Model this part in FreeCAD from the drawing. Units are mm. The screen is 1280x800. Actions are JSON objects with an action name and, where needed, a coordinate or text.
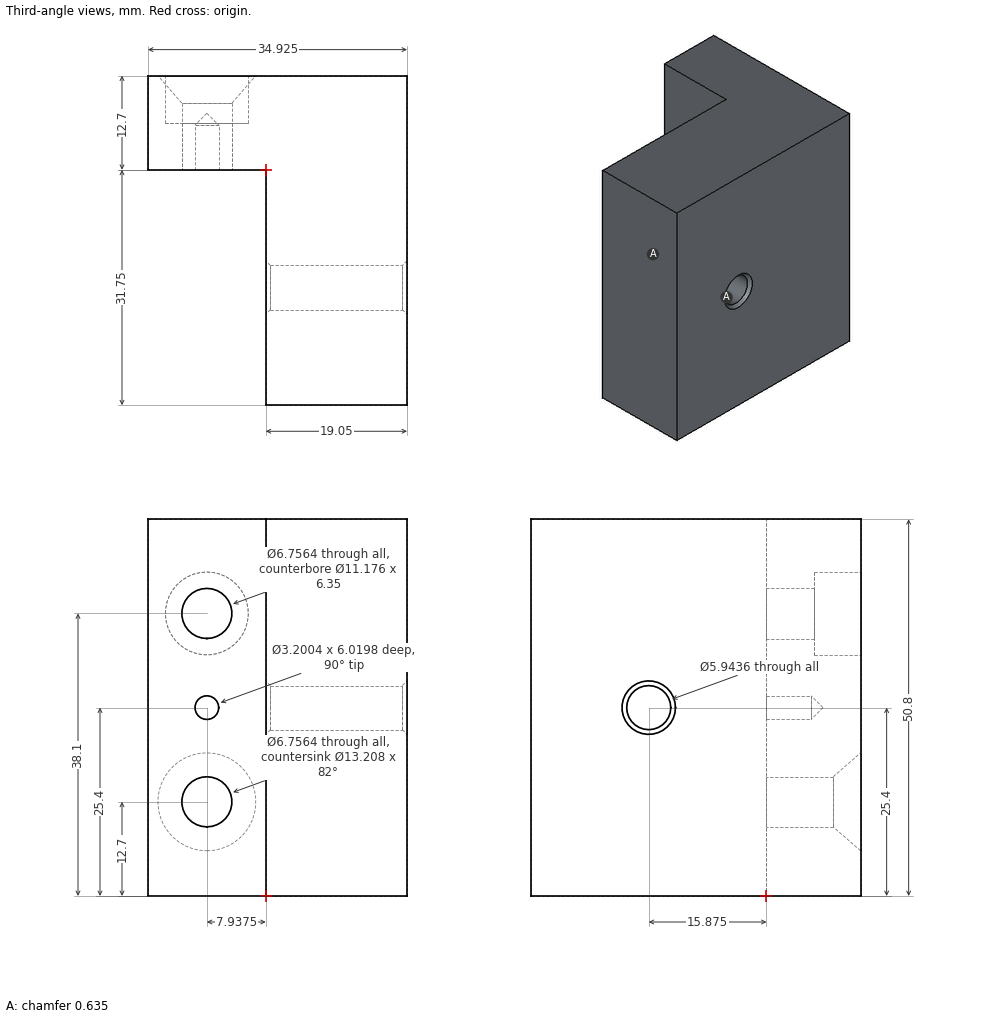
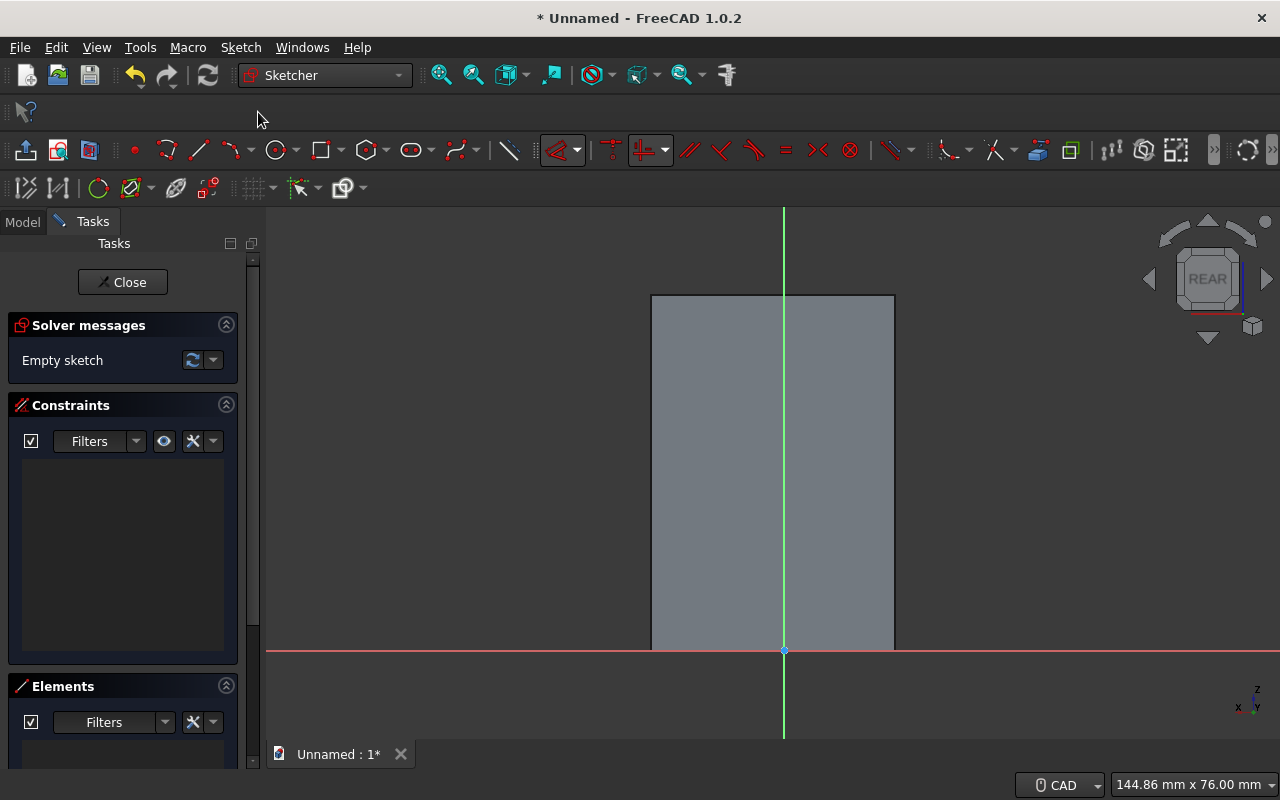
{"action": "scroll", "coordinate": [893, 665], "scroll_direction": "up", "scroll_amount": 5}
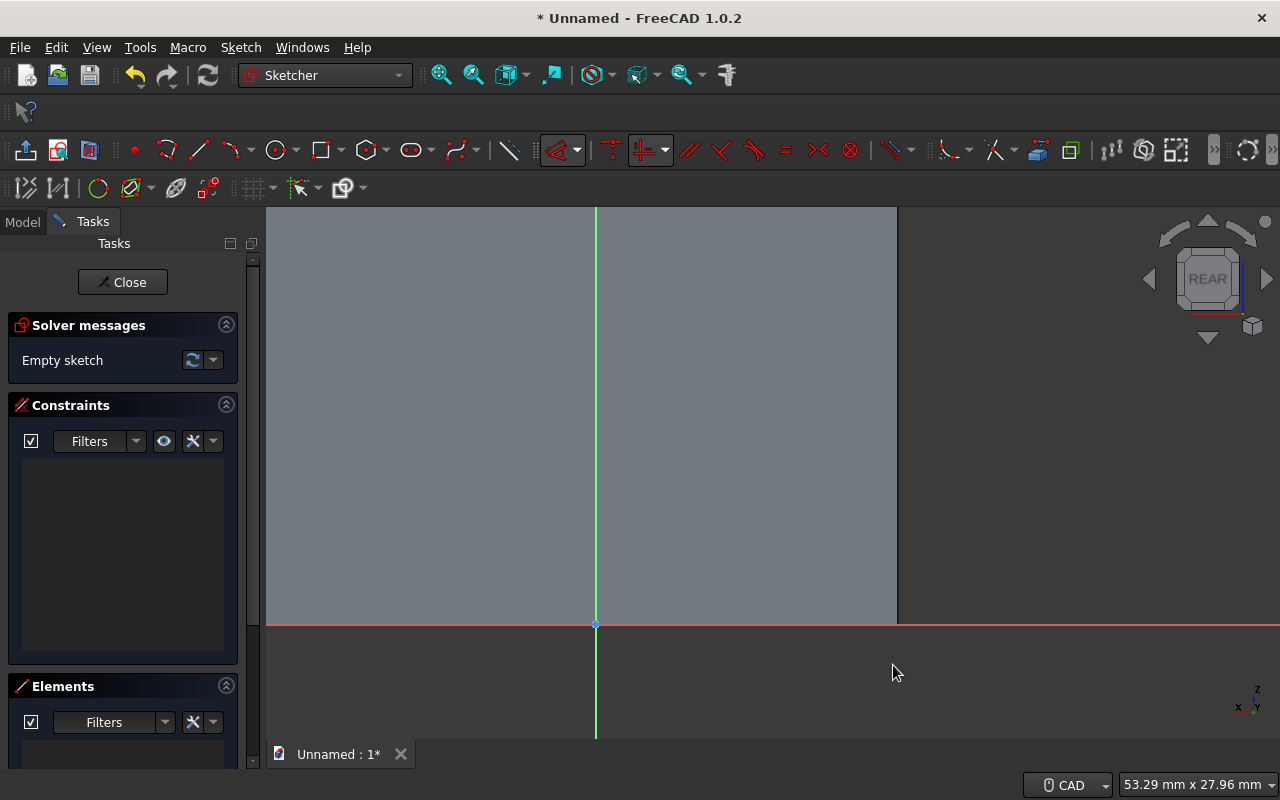
{"action": "left_click", "coordinate": [276, 150]}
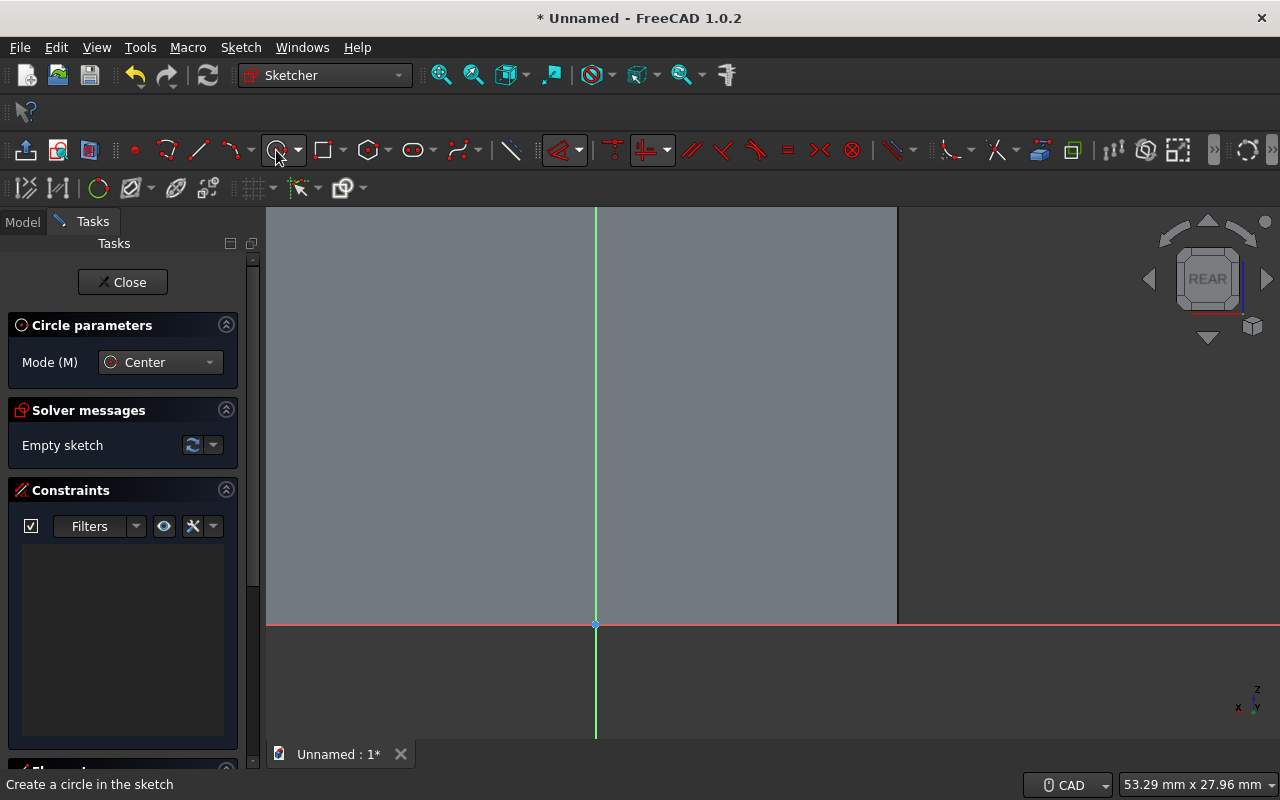
{"action": "left_click", "coordinate": [747, 383]}
{"action": "mouse_move", "coordinate": [792, 338]}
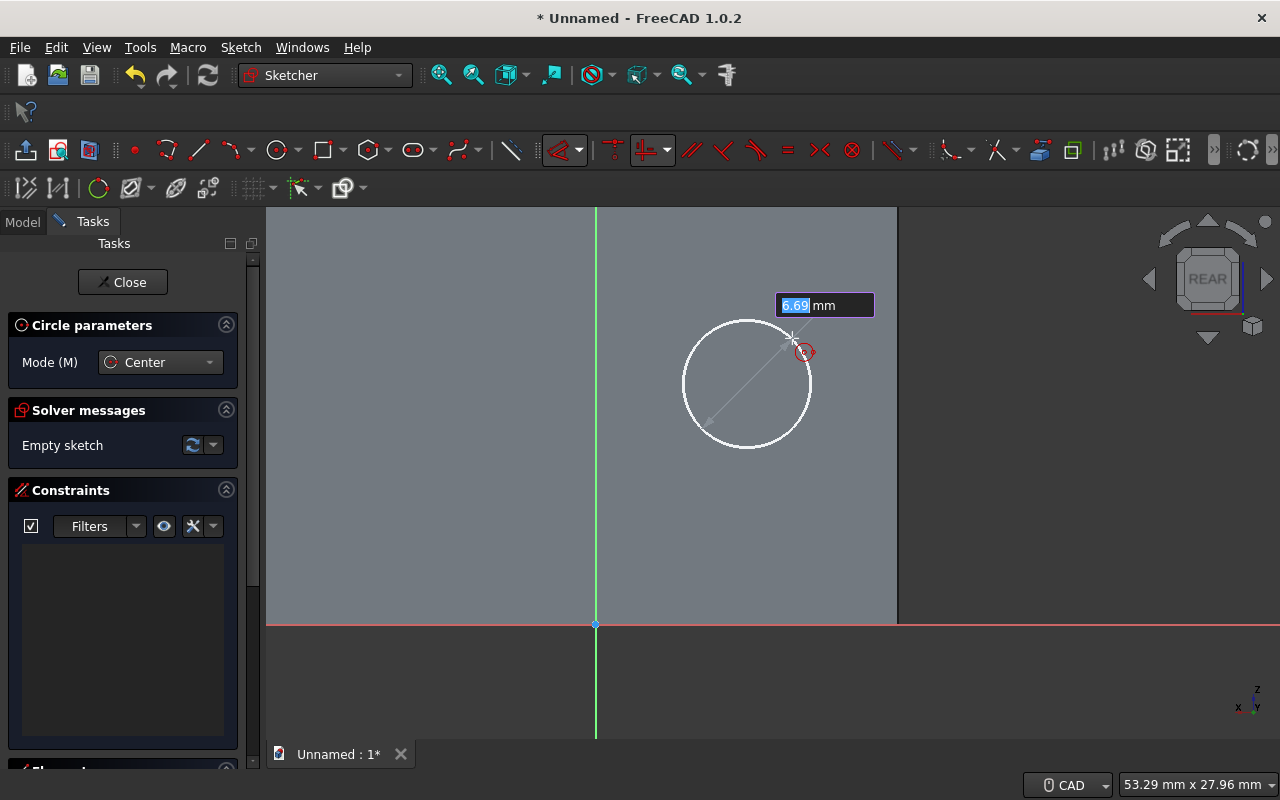
{"action": "type", "text": "6.7564"}
{"action": "key", "text": "Return"}
{"action": "key", "text": "Escape"}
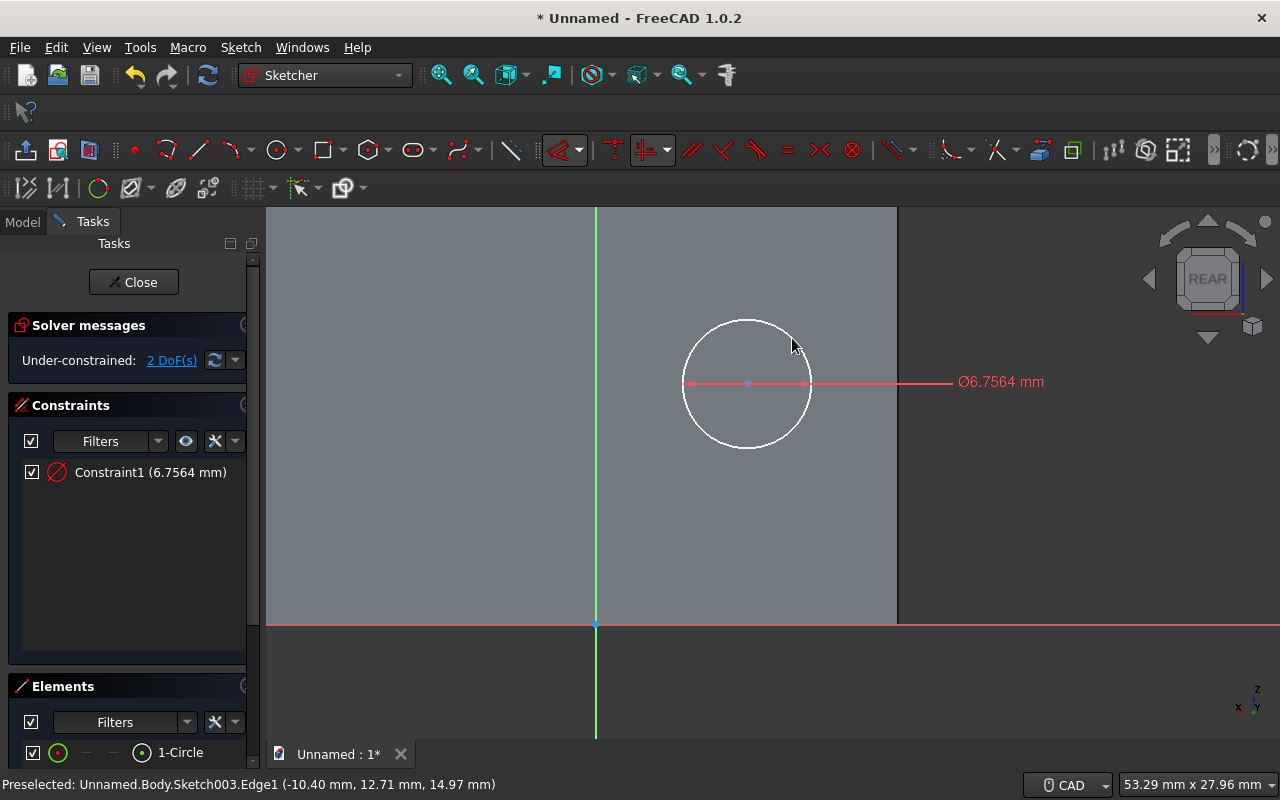
{"action": "left_click", "coordinate": [747, 384]}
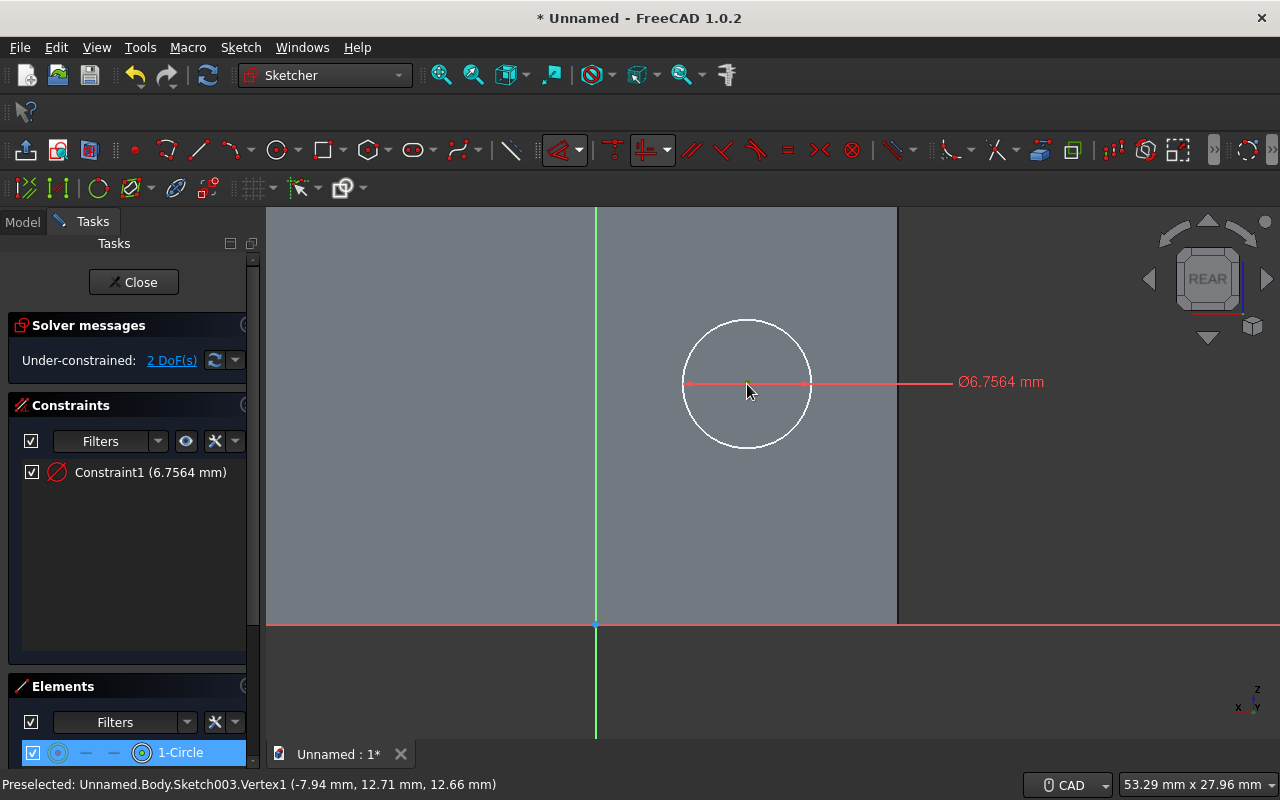
{"action": "left_click", "coordinate": [582, 150]}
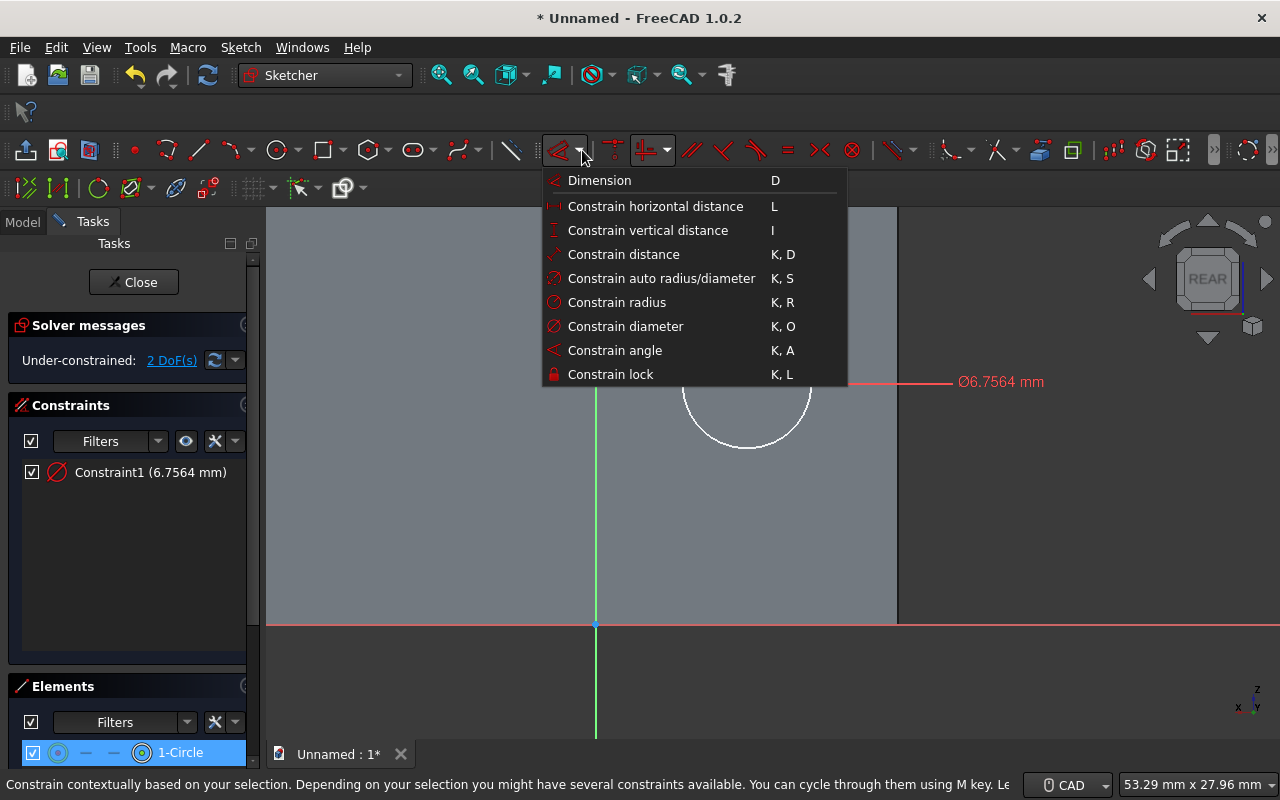
{"action": "left_click", "coordinate": [695, 230]}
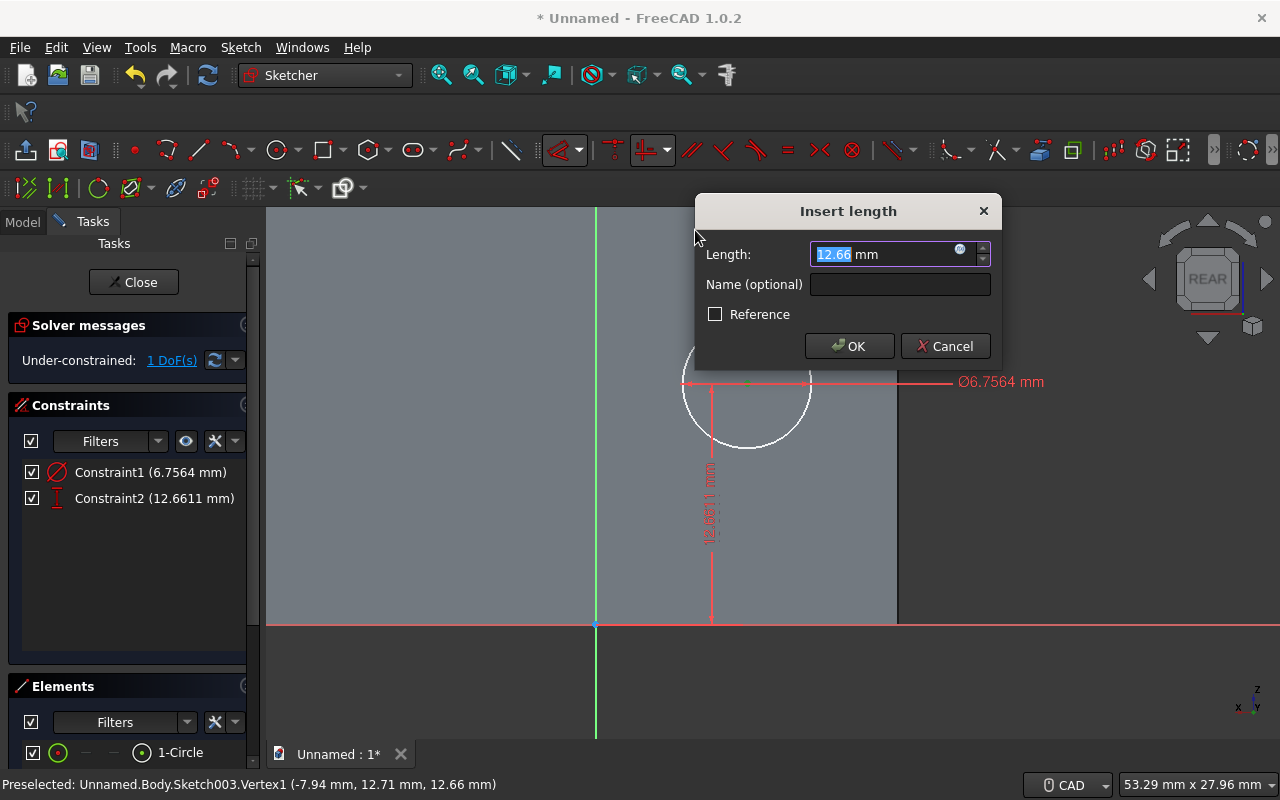
{"action": "type", "text": "12.7"}
{"action": "key", "text": "Return"}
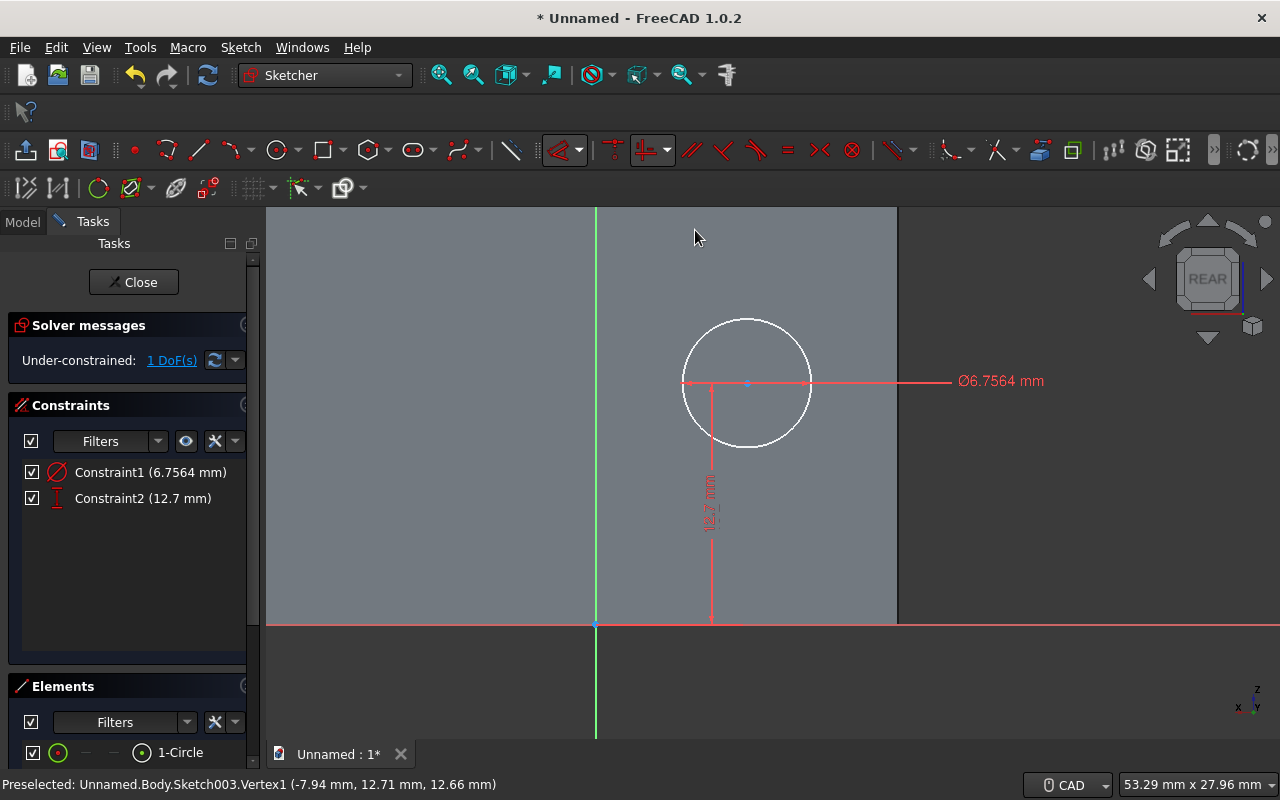
{"action": "left_click", "coordinate": [747, 383]}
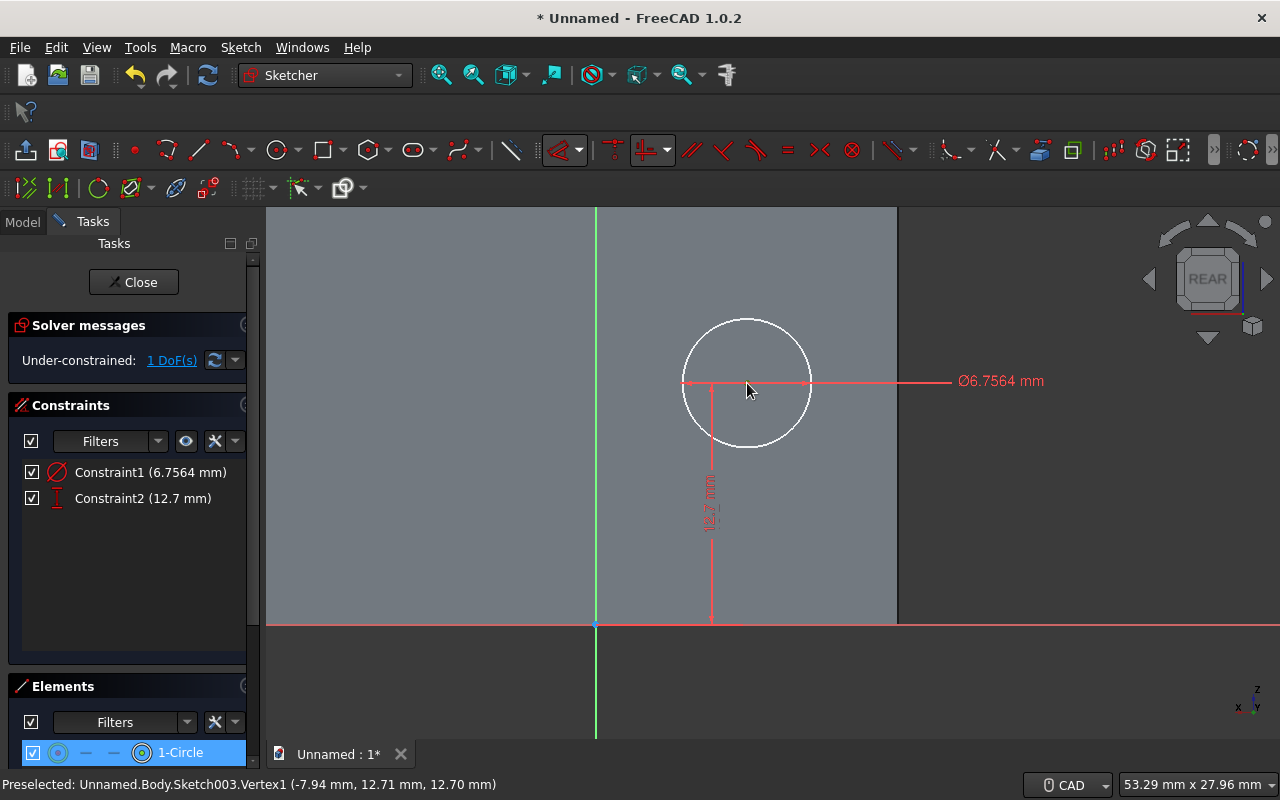
{"action": "left_click", "coordinate": [582, 150]}